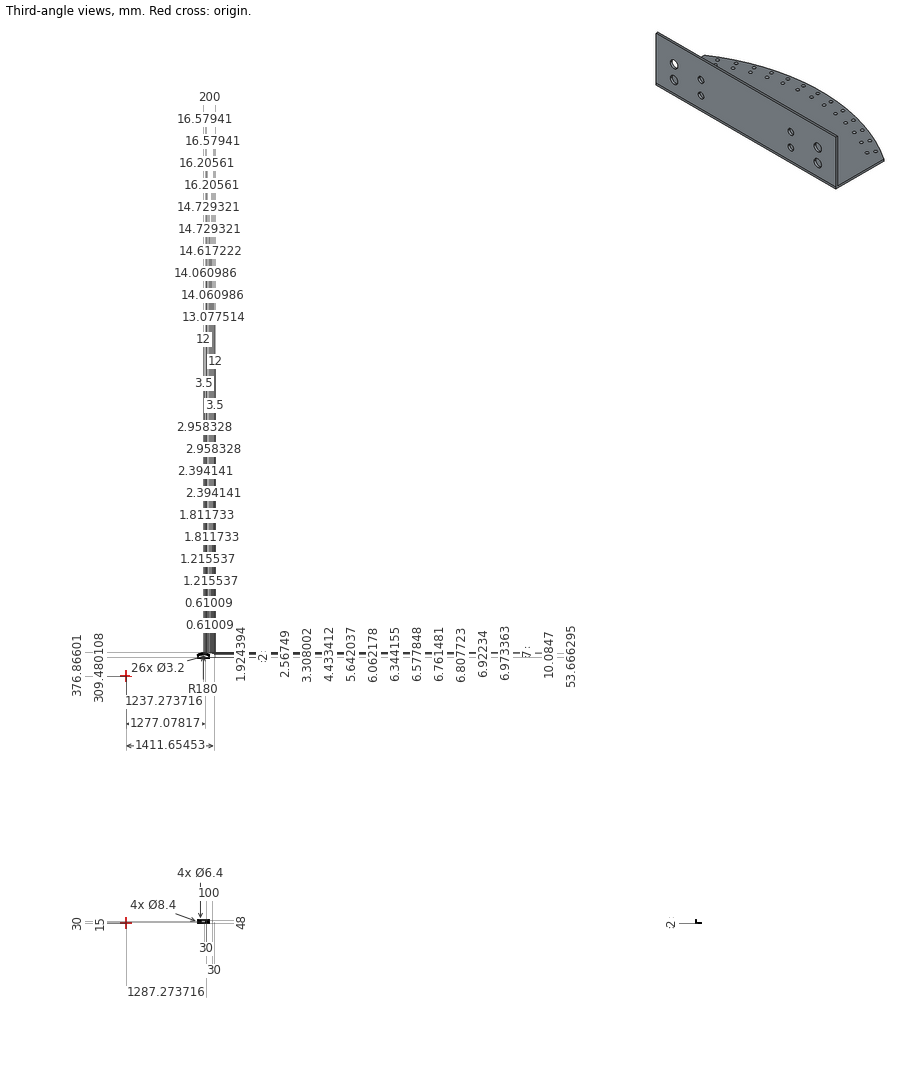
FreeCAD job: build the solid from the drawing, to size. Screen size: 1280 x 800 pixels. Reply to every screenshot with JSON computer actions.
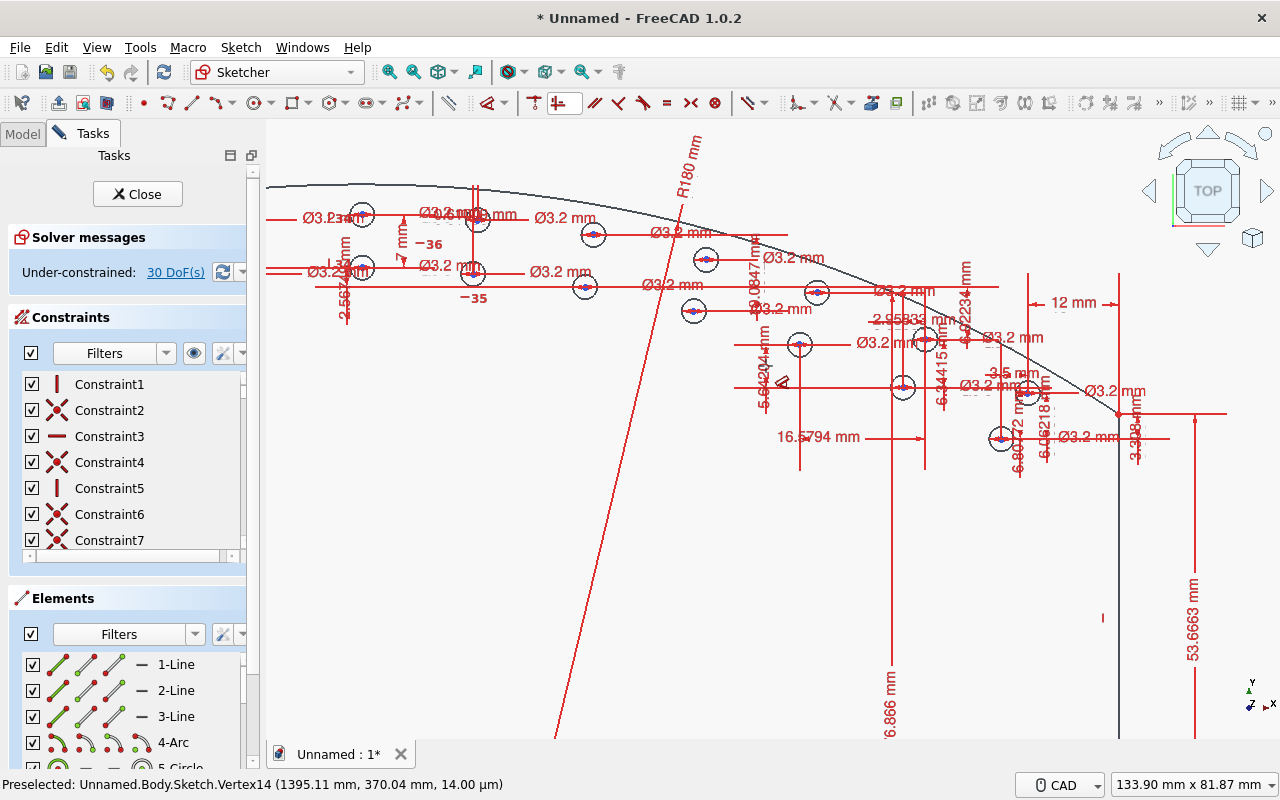
{"action": "scroll", "coordinate": [904, 388], "scroll_direction": "down", "scroll_amount": 5}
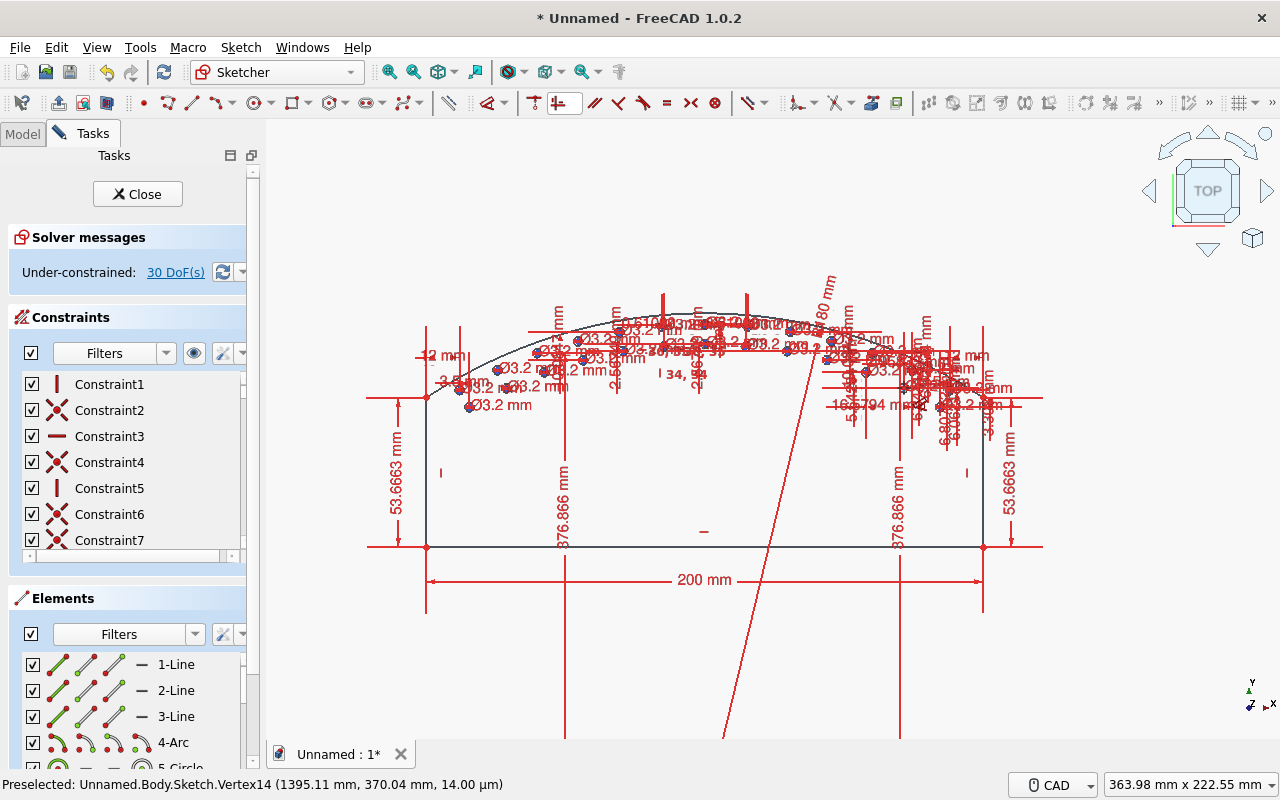
{"action": "scroll", "coordinate": [426, 398], "scroll_direction": "up", "scroll_amount": 8}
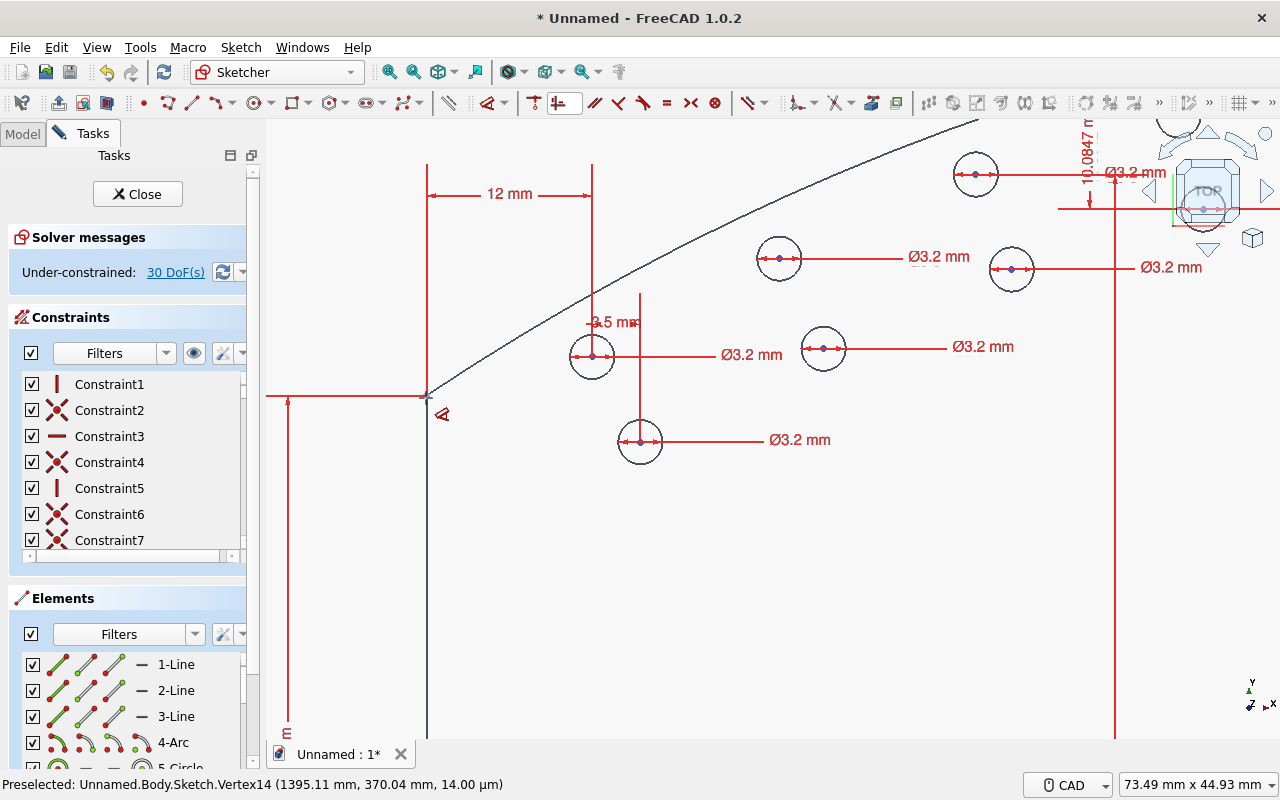
{"action": "left_click", "coordinate": [427, 396]}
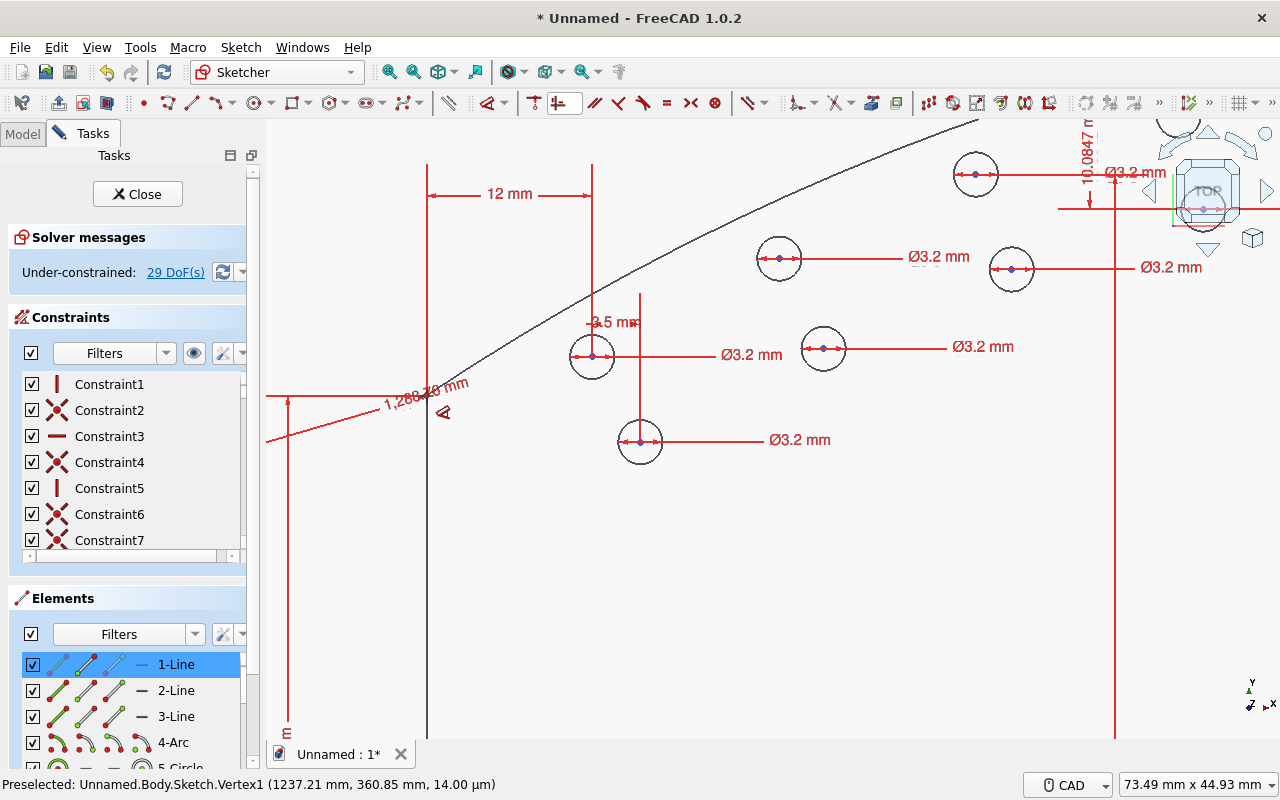
{"action": "left_click", "coordinate": [640, 442]}
{"action": "left_click", "coordinate": [393, 419]}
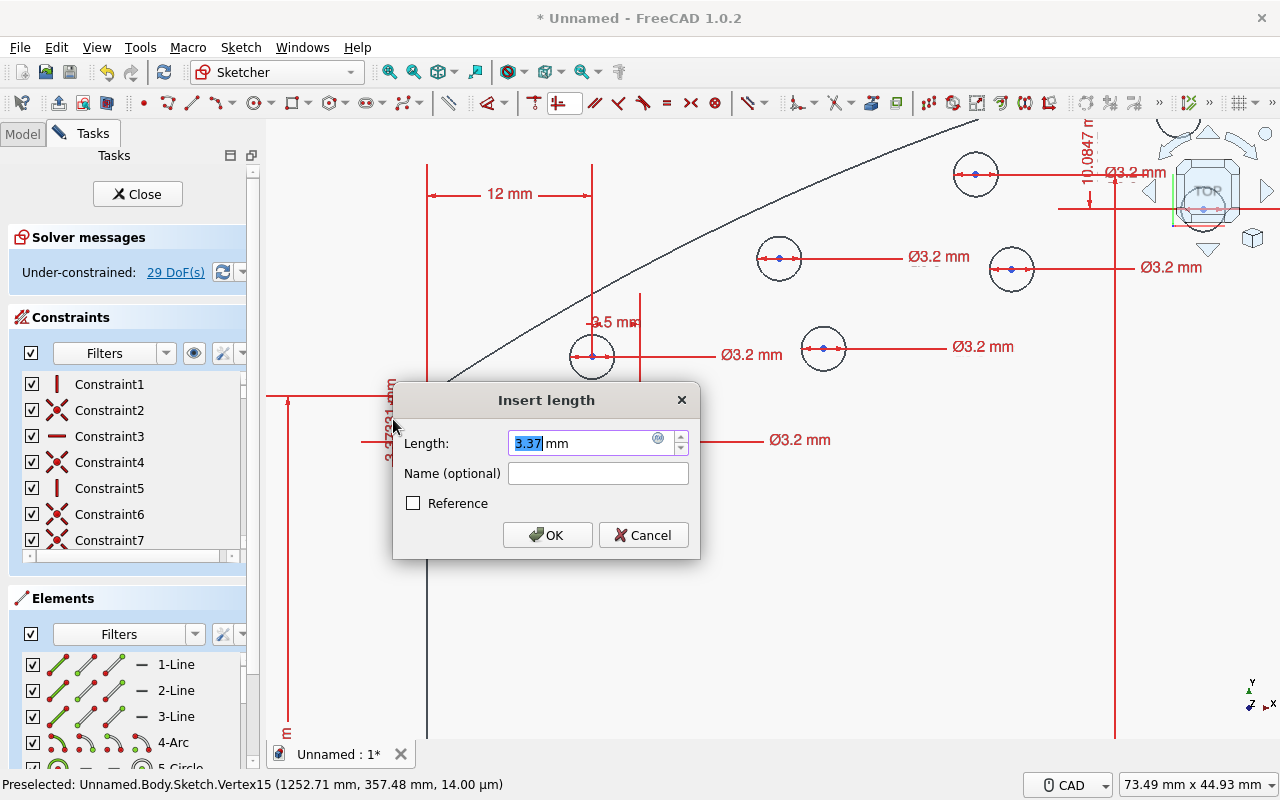
{"action": "type", "text": "3.308002"}
{"action": "key", "text": "Return"}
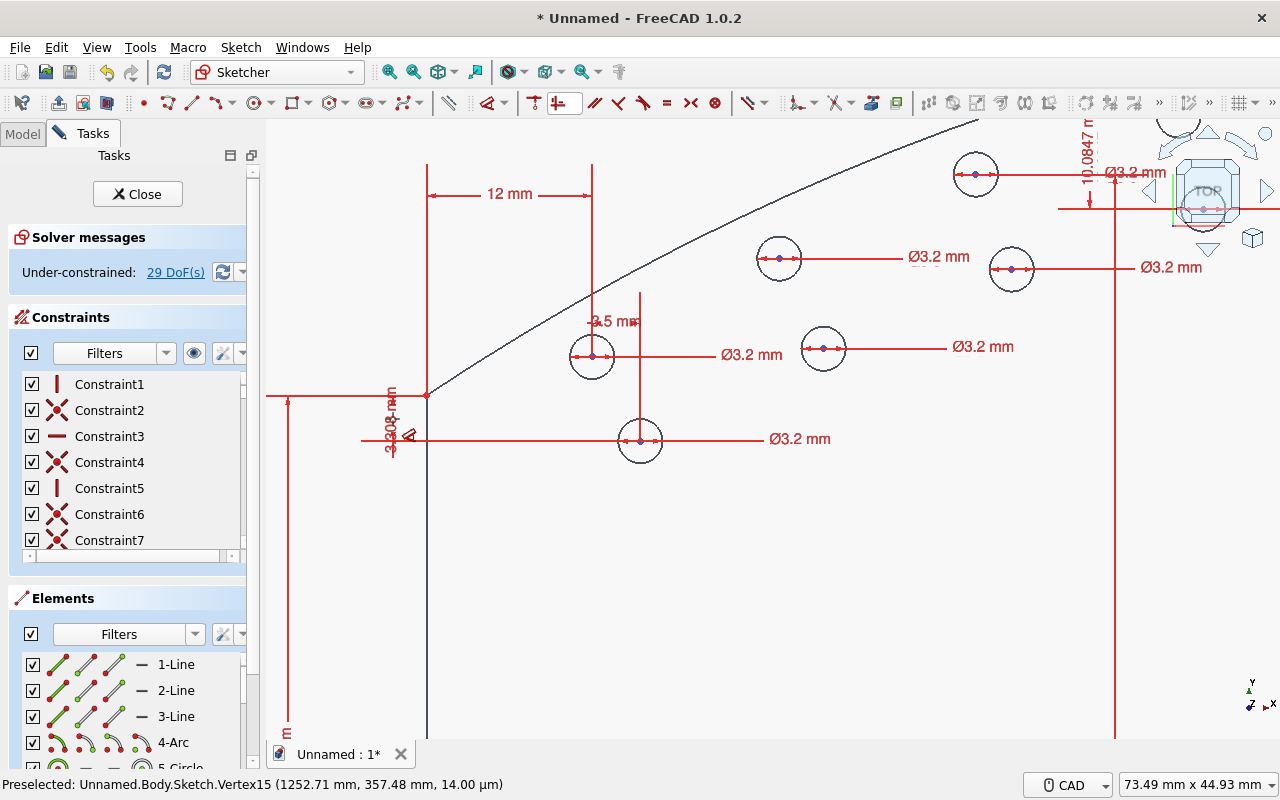
{"action": "left_click", "coordinate": [640, 441]}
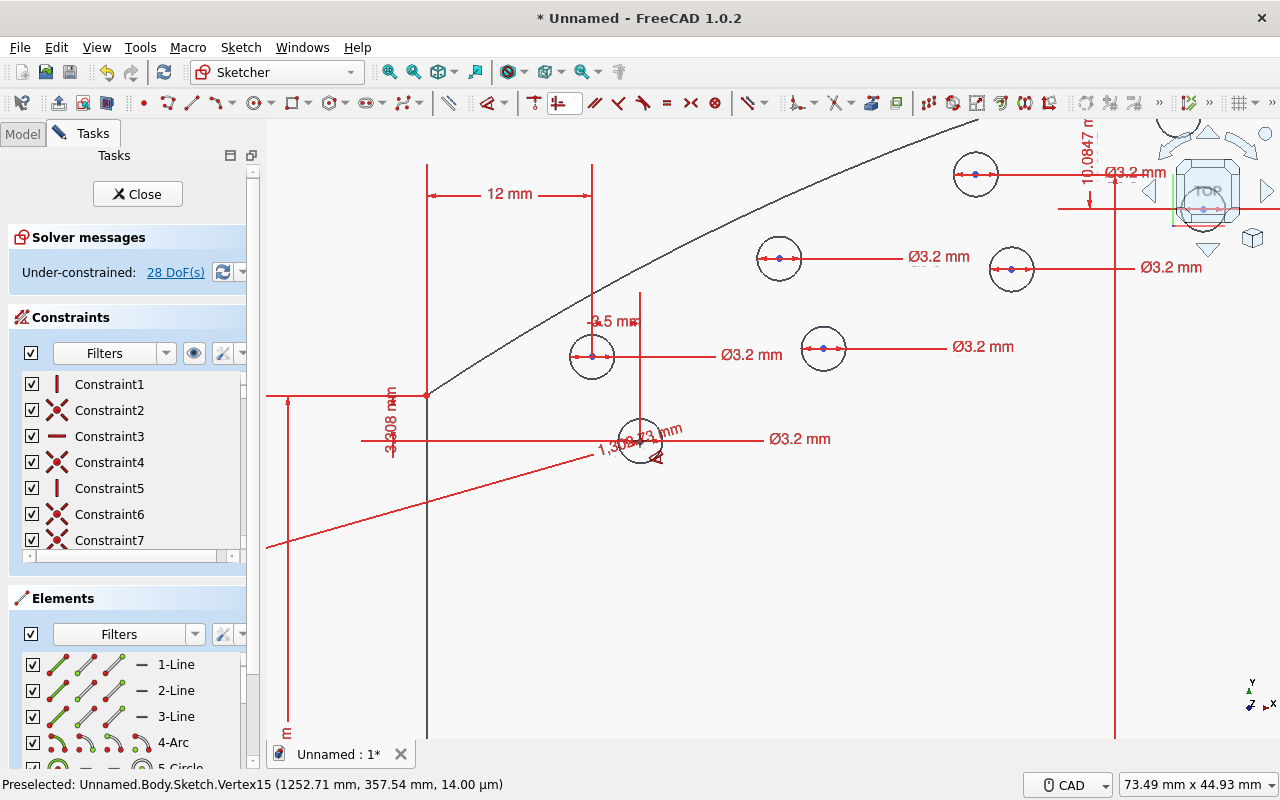
{"action": "left_click", "coordinate": [592, 357]}
{"action": "left_click", "coordinate": [558, 399]}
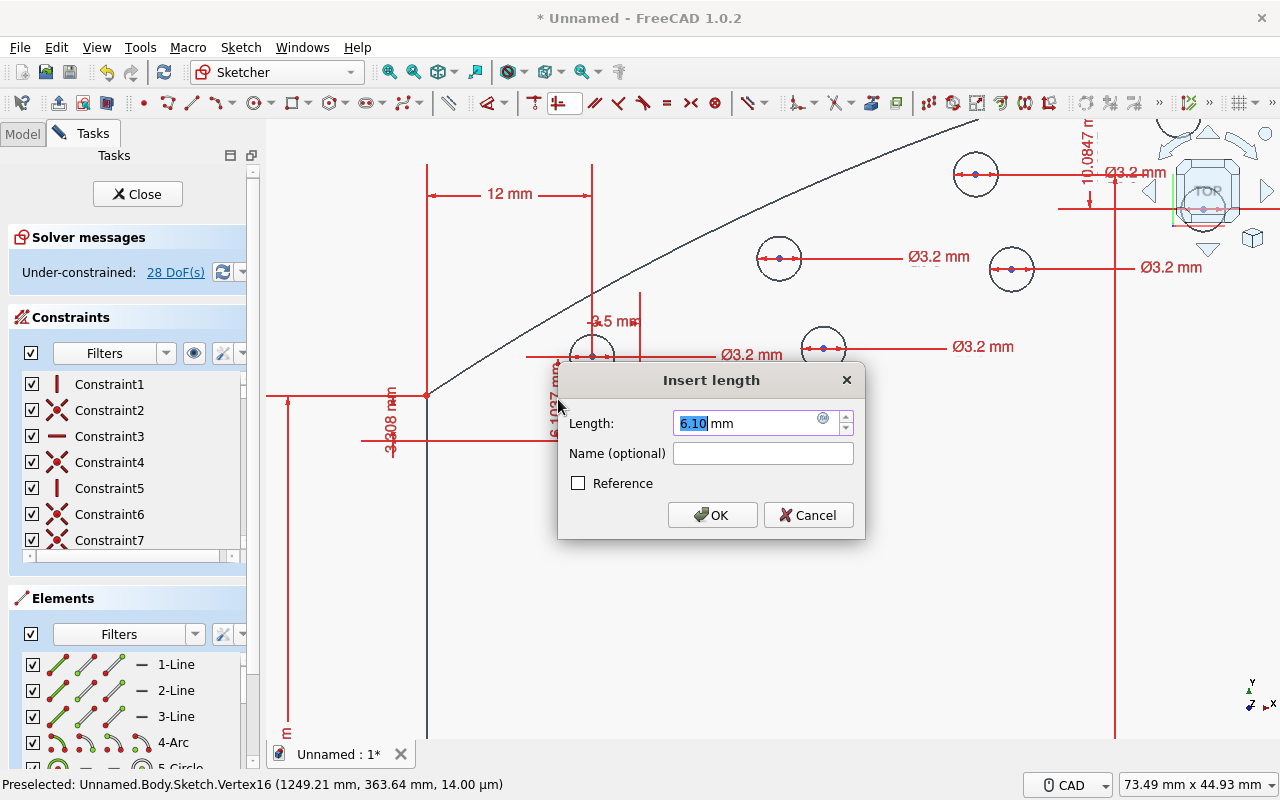
{"action": "type", "text": "6.062178"}
{"action": "key", "text": "Return"}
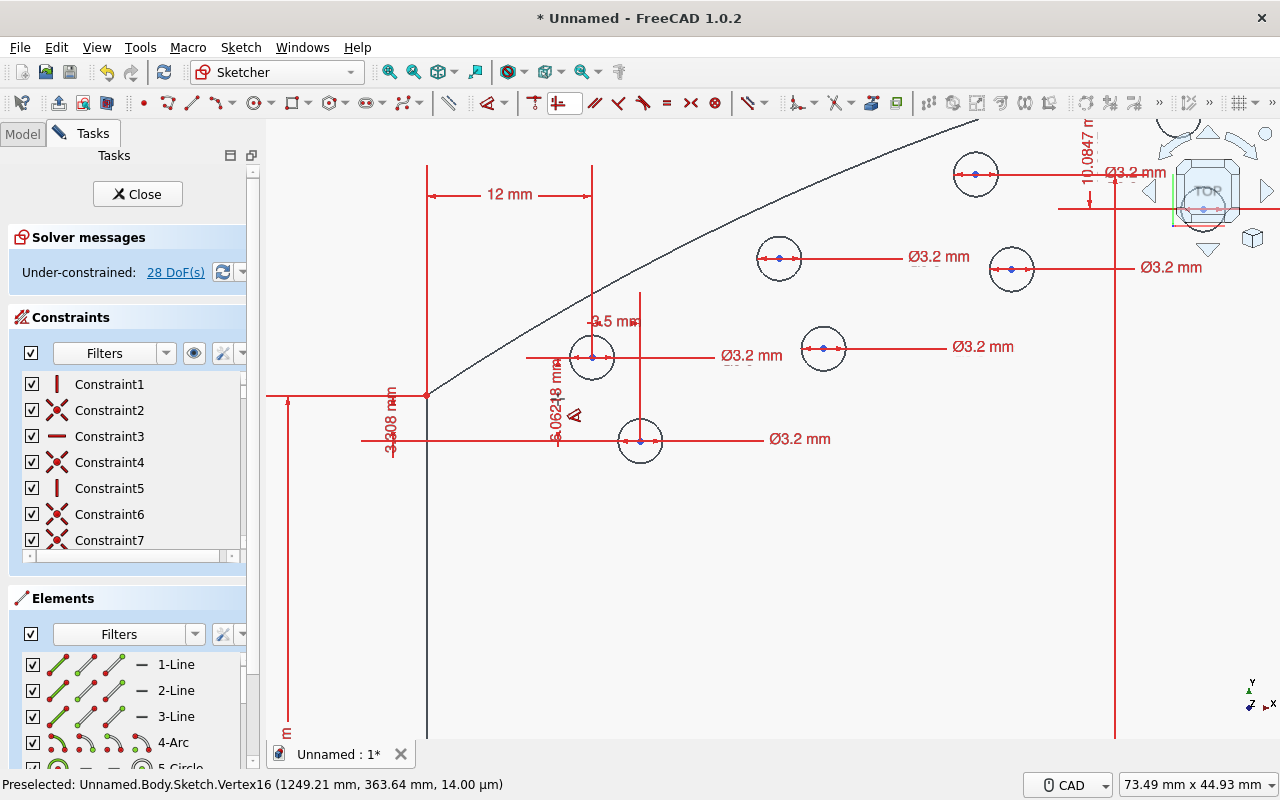
{"action": "left_click", "coordinate": [640, 441]}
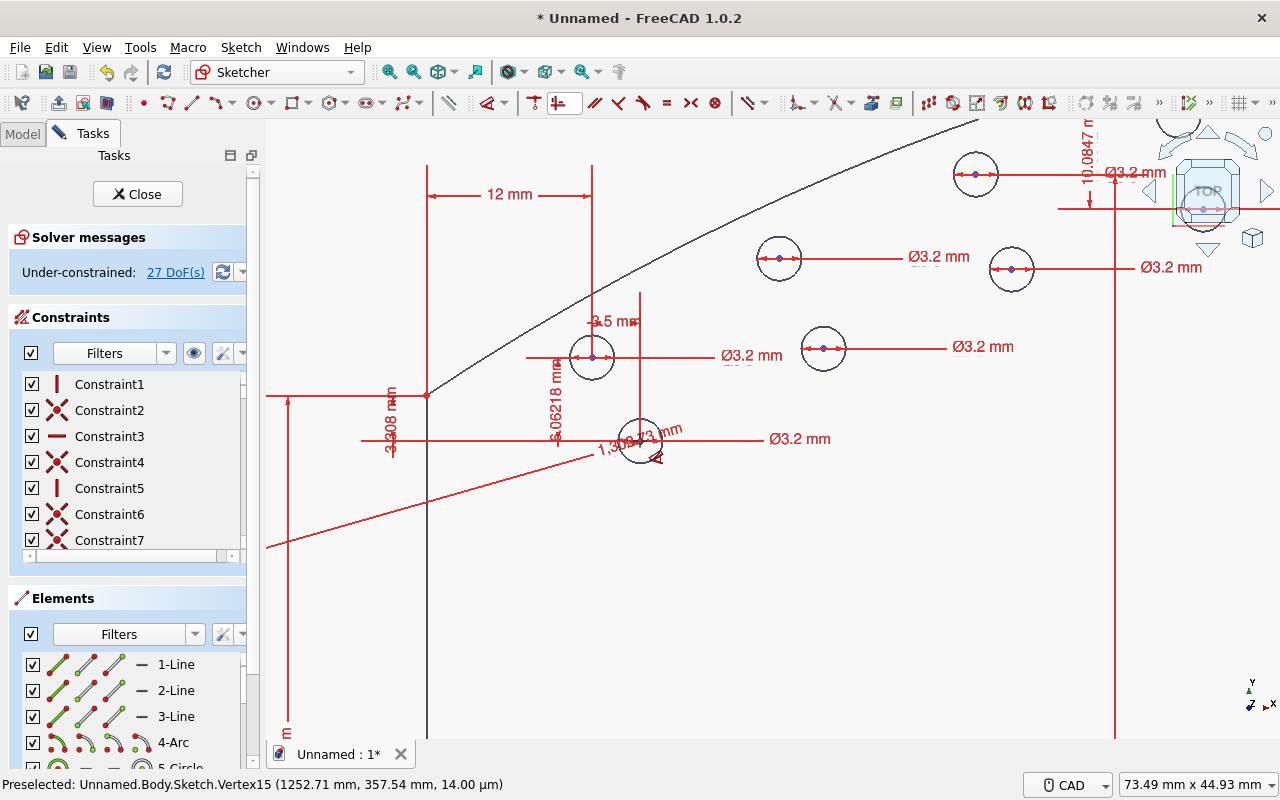
{"action": "left_click", "coordinate": [824, 349]}
{"action": "left_click", "coordinate": [606, 427]}